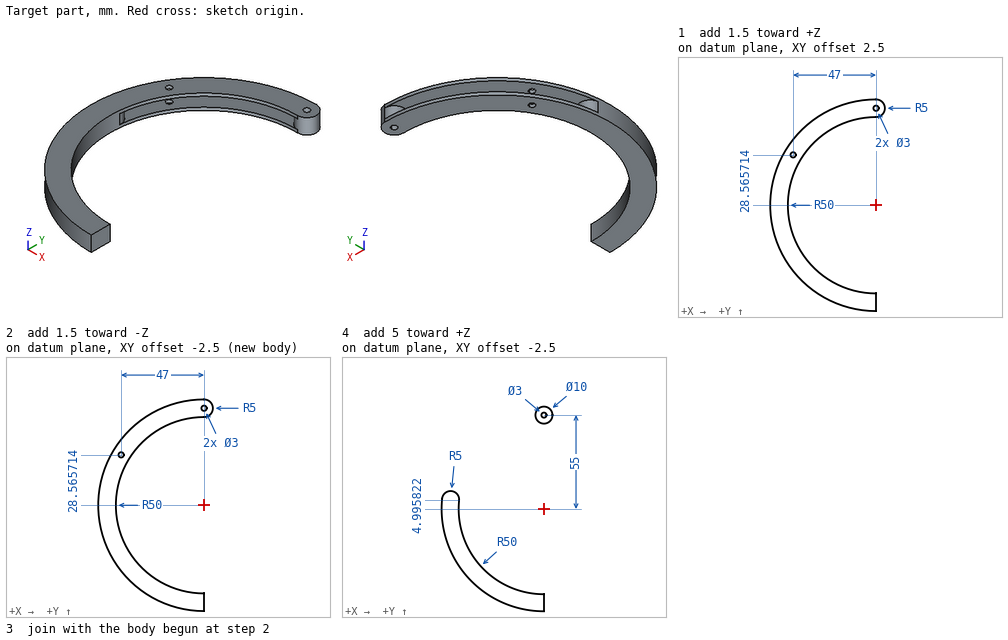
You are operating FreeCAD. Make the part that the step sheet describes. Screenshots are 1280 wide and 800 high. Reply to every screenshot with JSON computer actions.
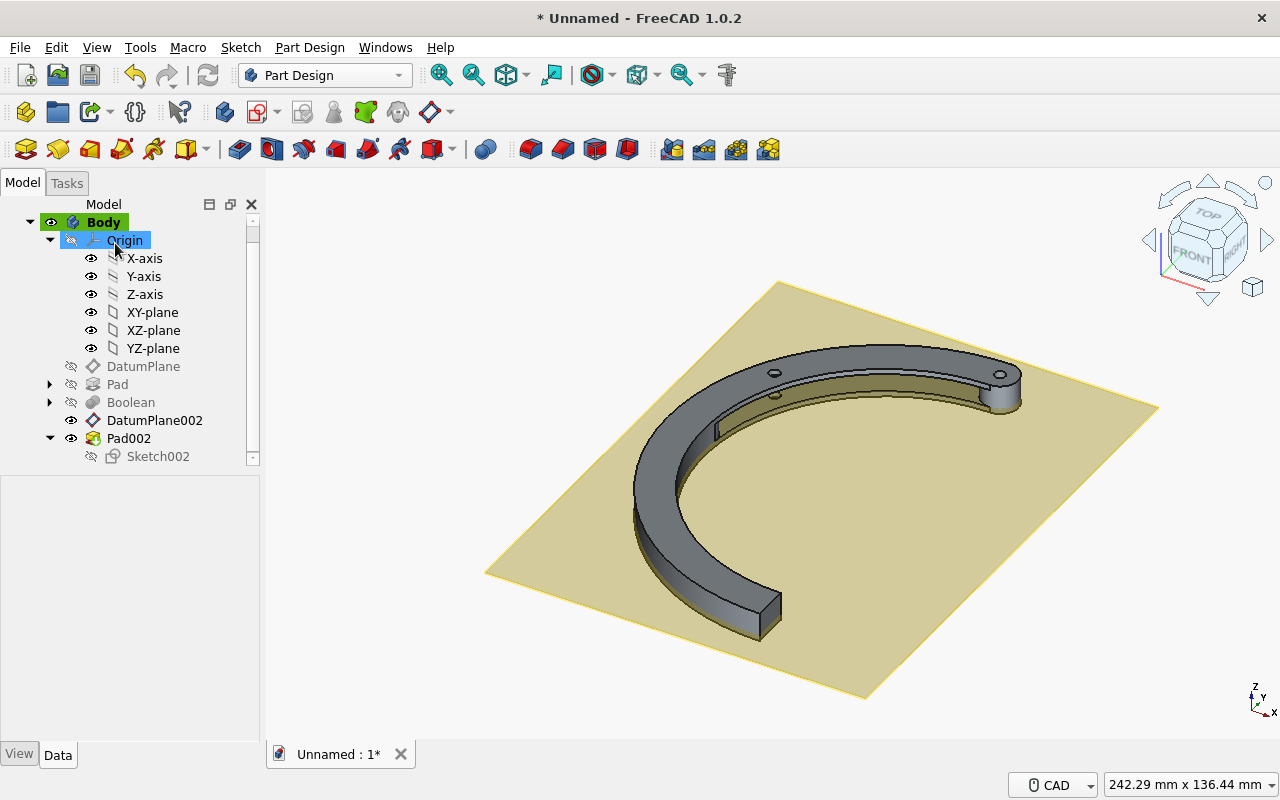
{"action": "left_click", "coordinate": [116, 420]}
{"action": "key", "text": "space"}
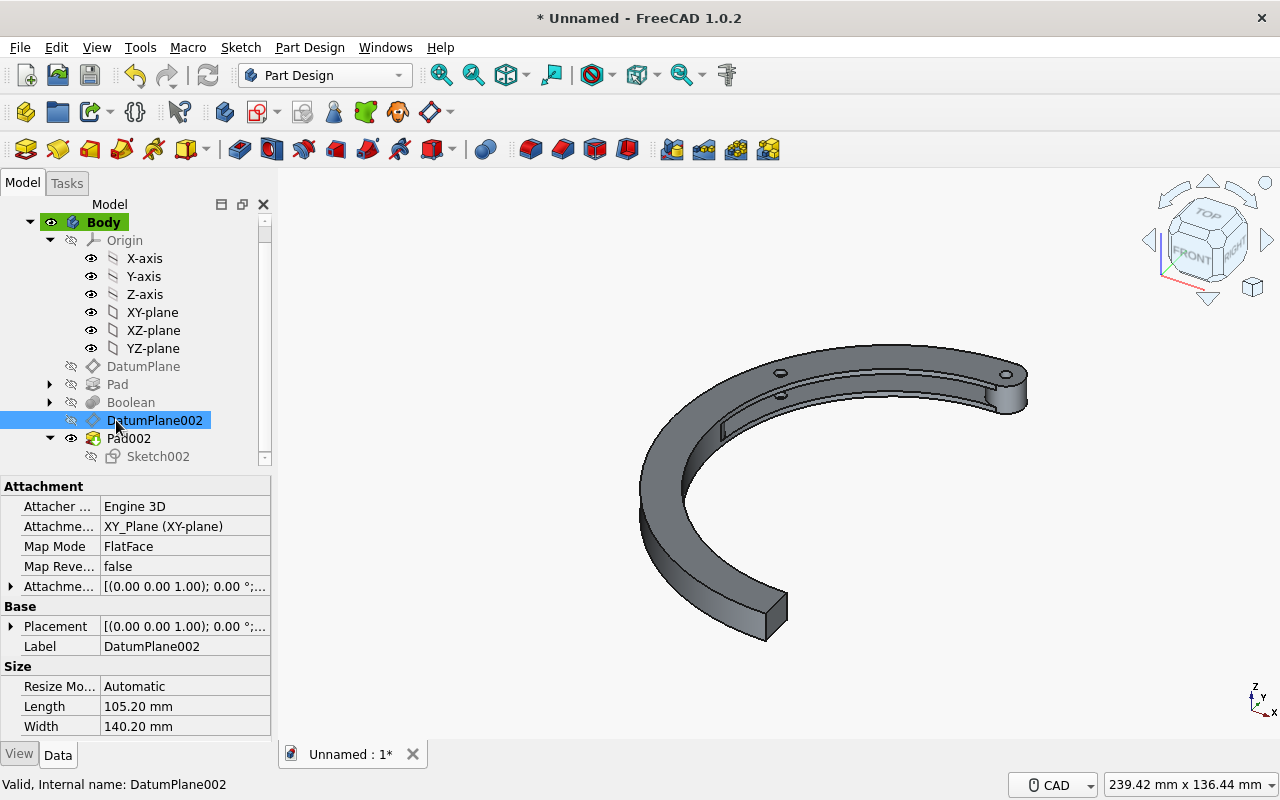
{"action": "key", "text": "0"}